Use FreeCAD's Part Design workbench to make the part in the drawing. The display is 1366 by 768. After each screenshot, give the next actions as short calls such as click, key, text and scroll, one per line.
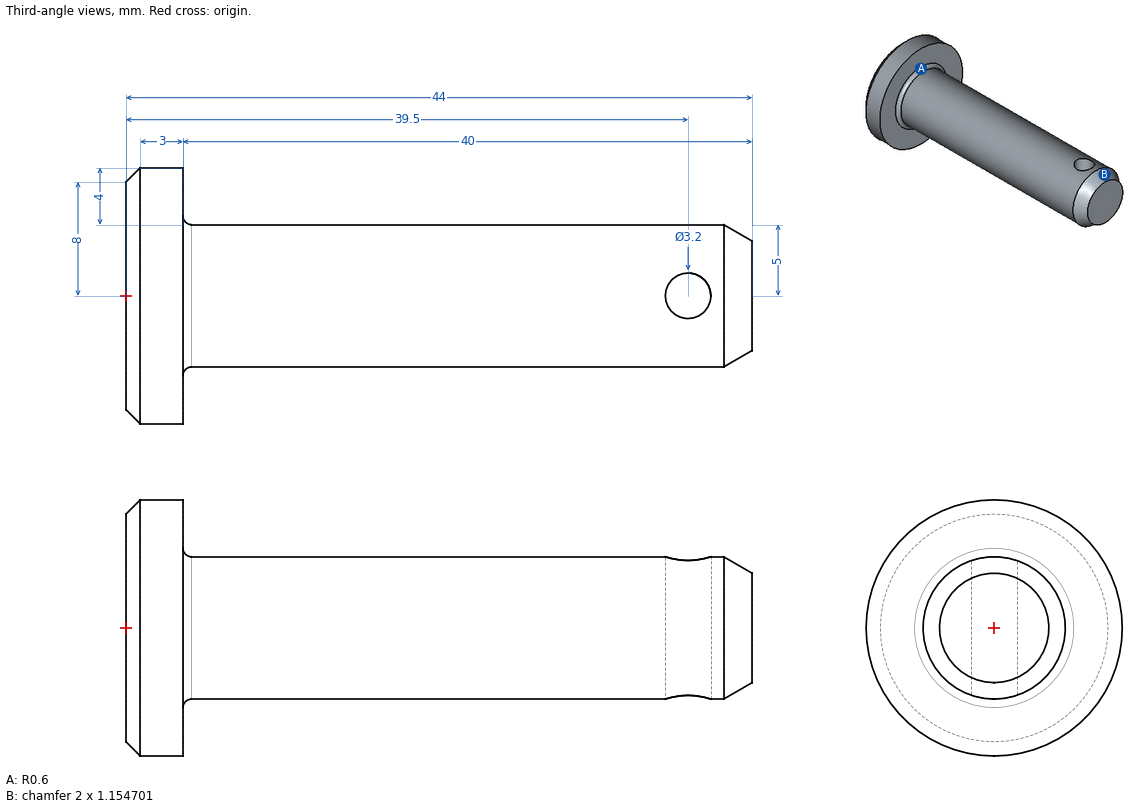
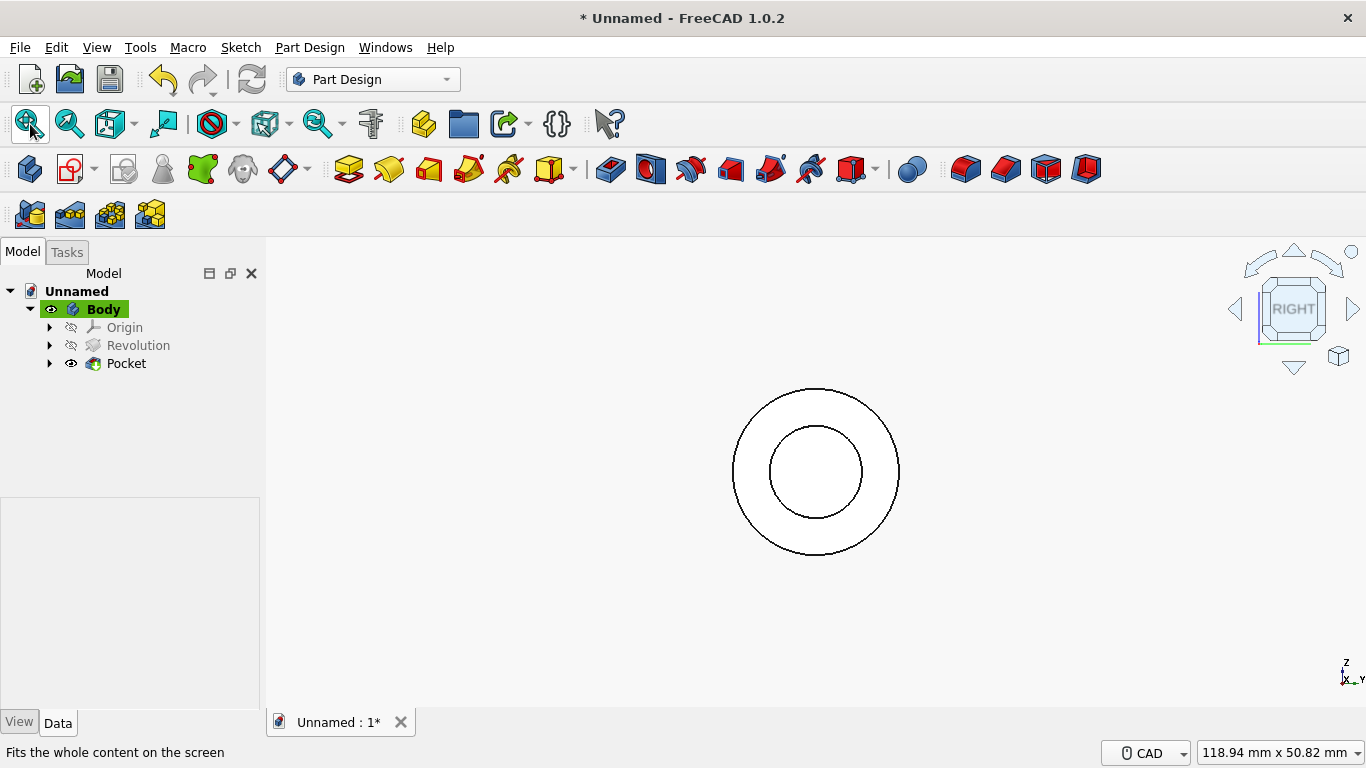
key(5)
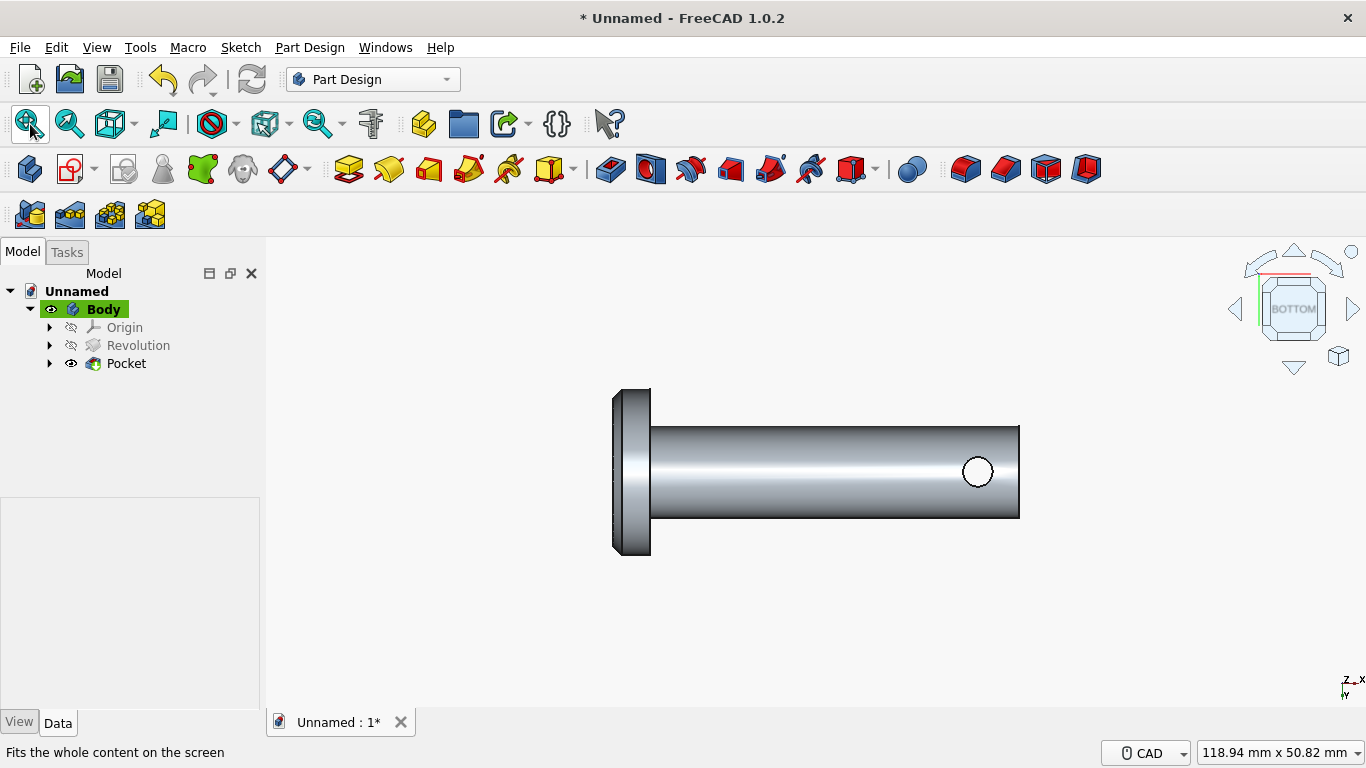
click(30, 124)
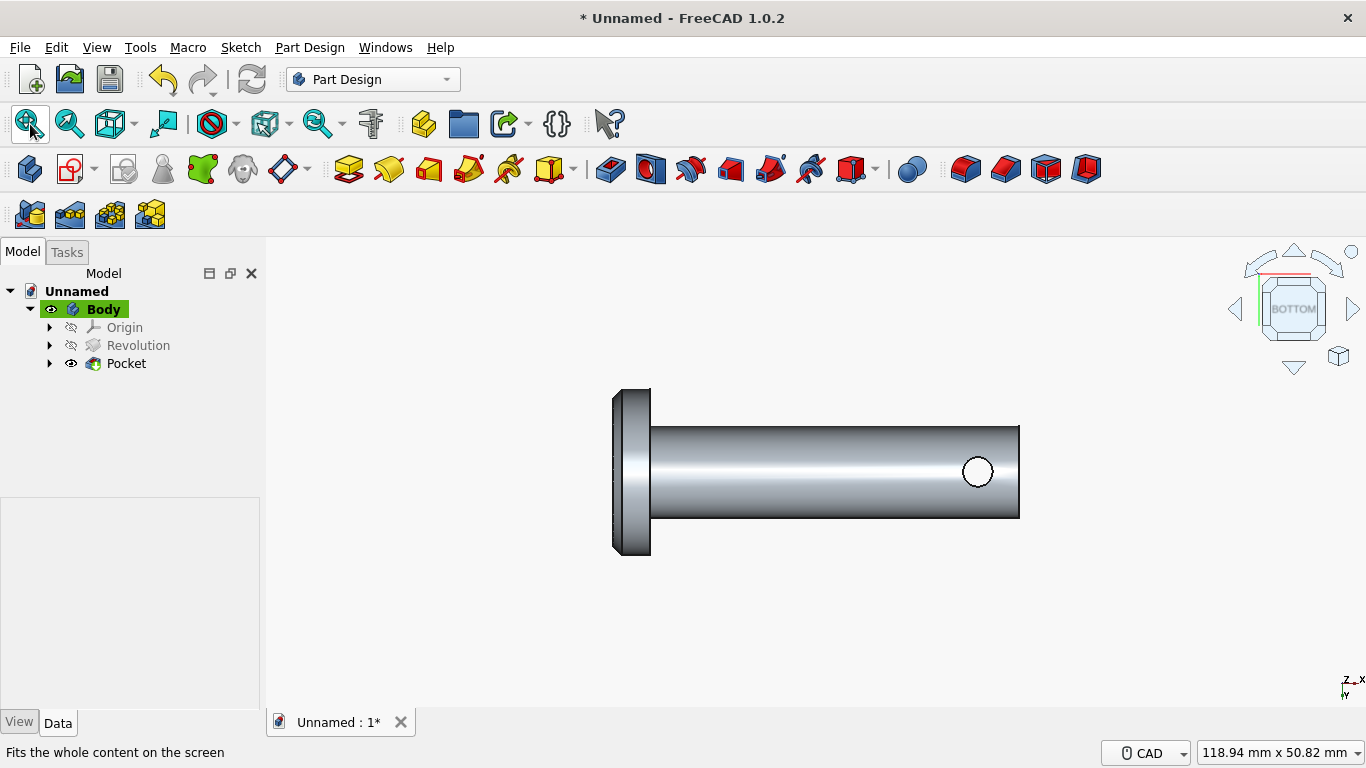
key(4)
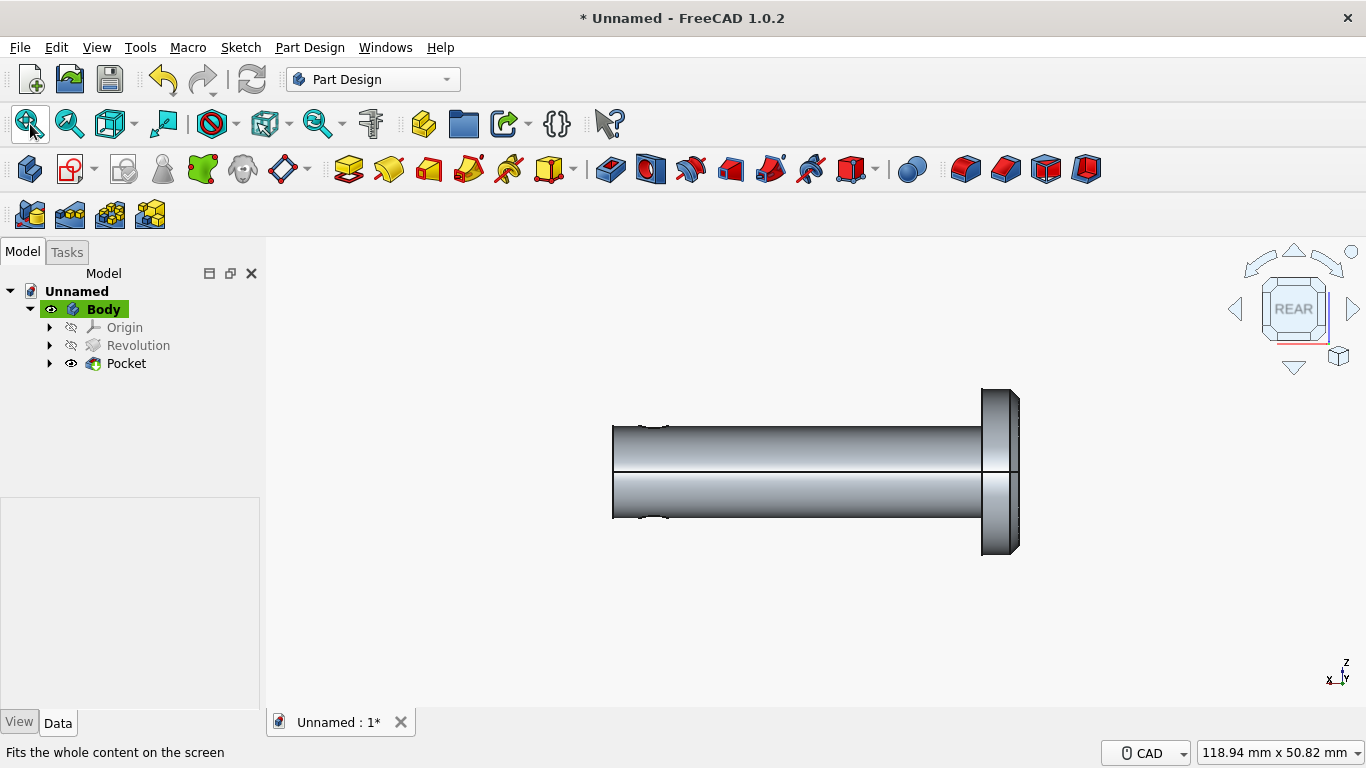
click(30, 124)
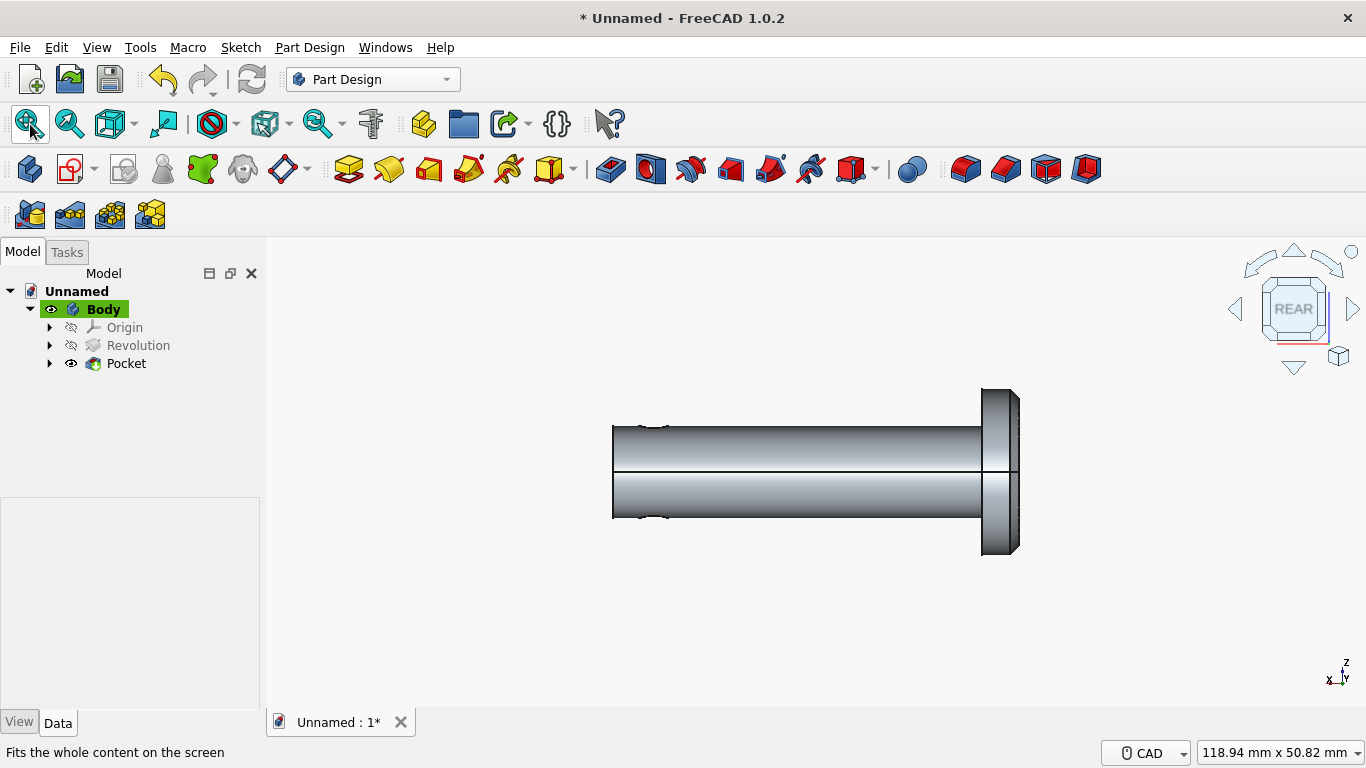
key(6)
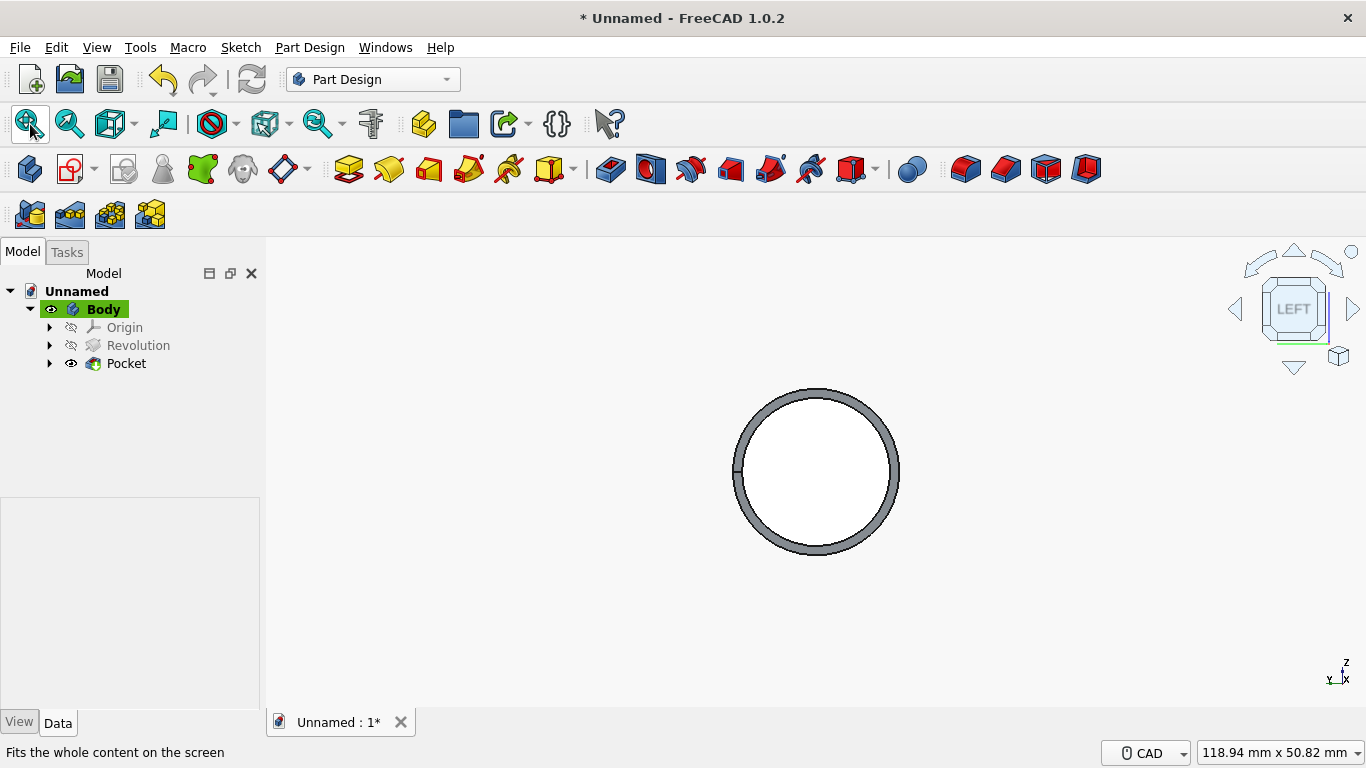
click(30, 124)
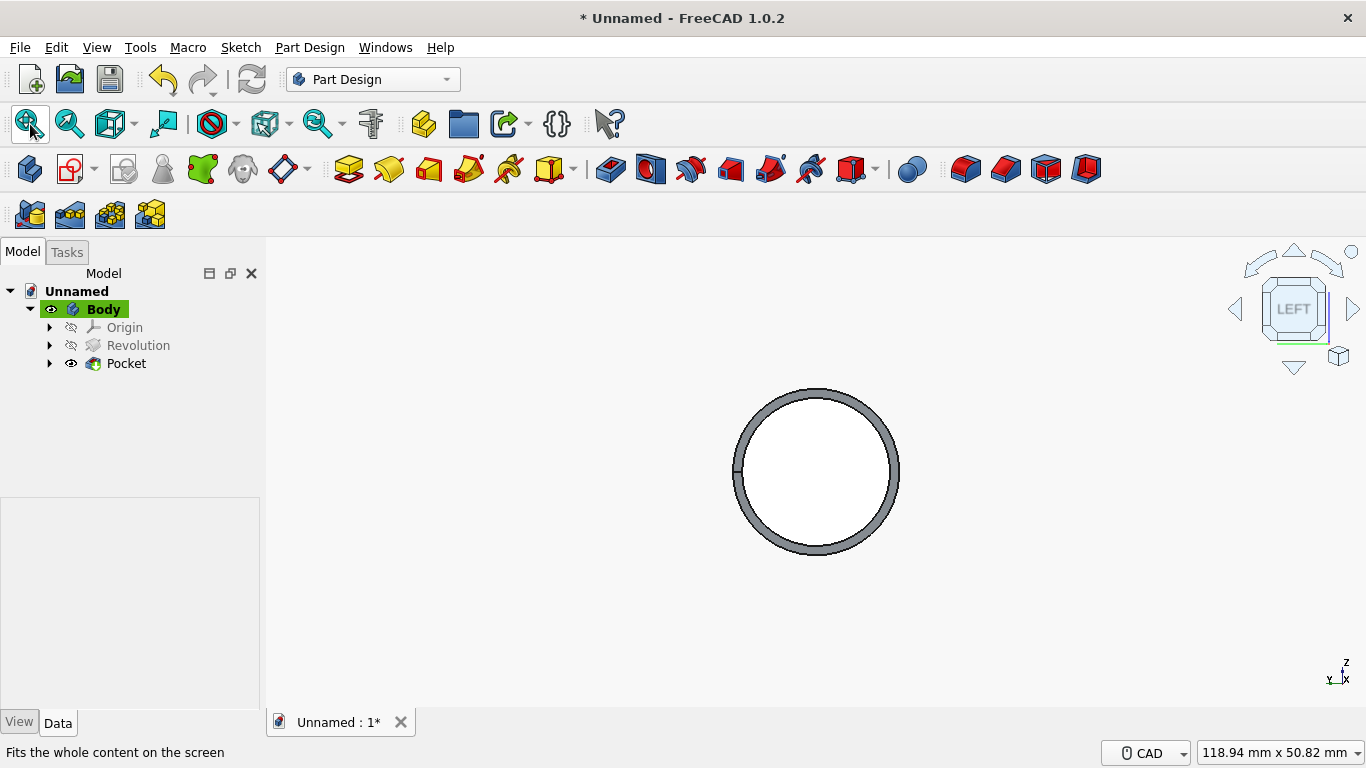
key(v)
key(3)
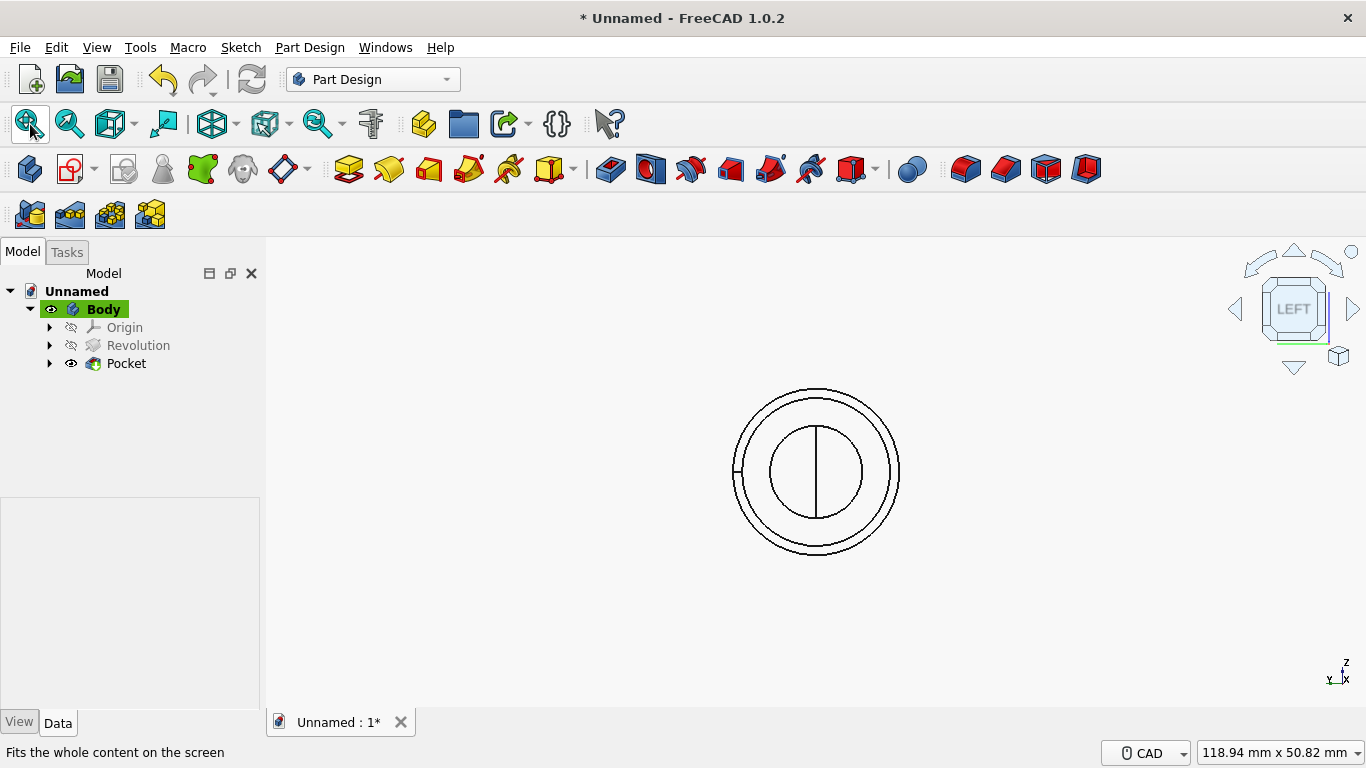
key(0)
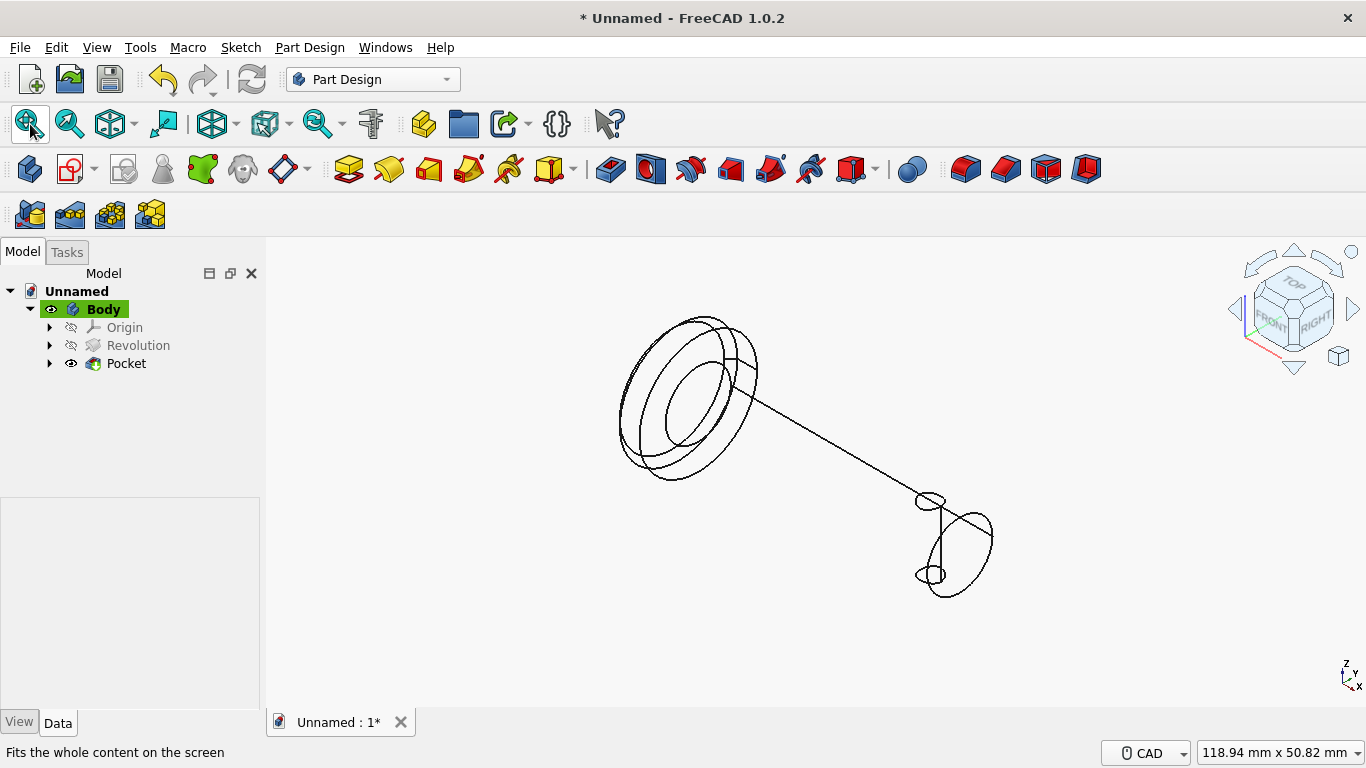
click(666, 422)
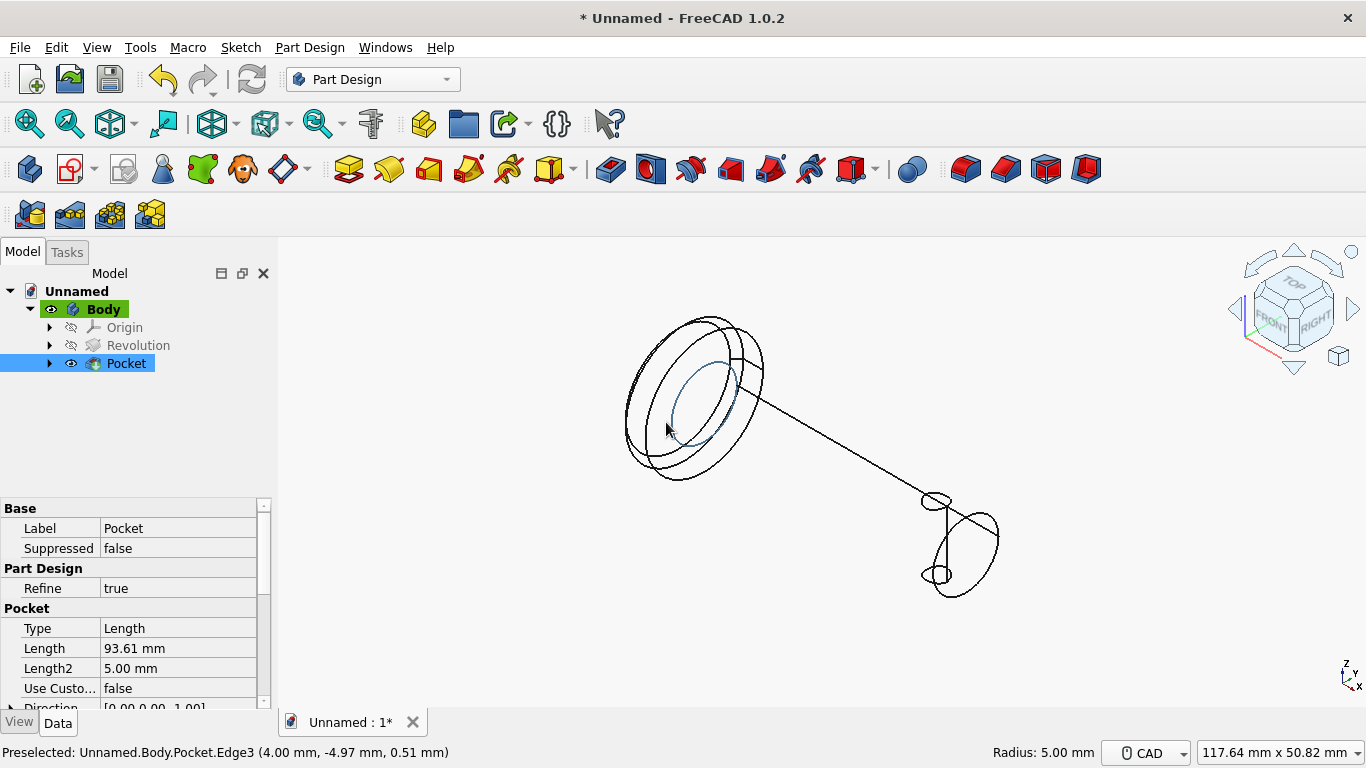
key(v)
key(1)